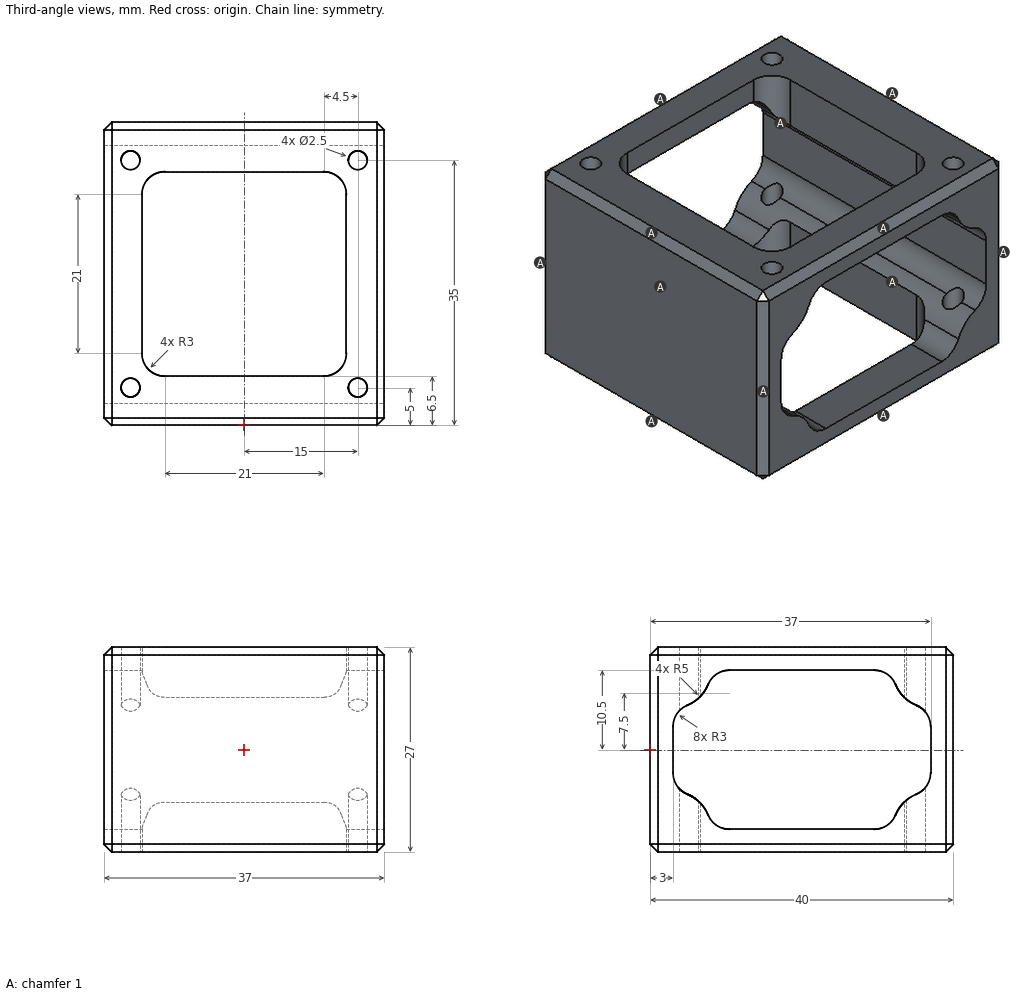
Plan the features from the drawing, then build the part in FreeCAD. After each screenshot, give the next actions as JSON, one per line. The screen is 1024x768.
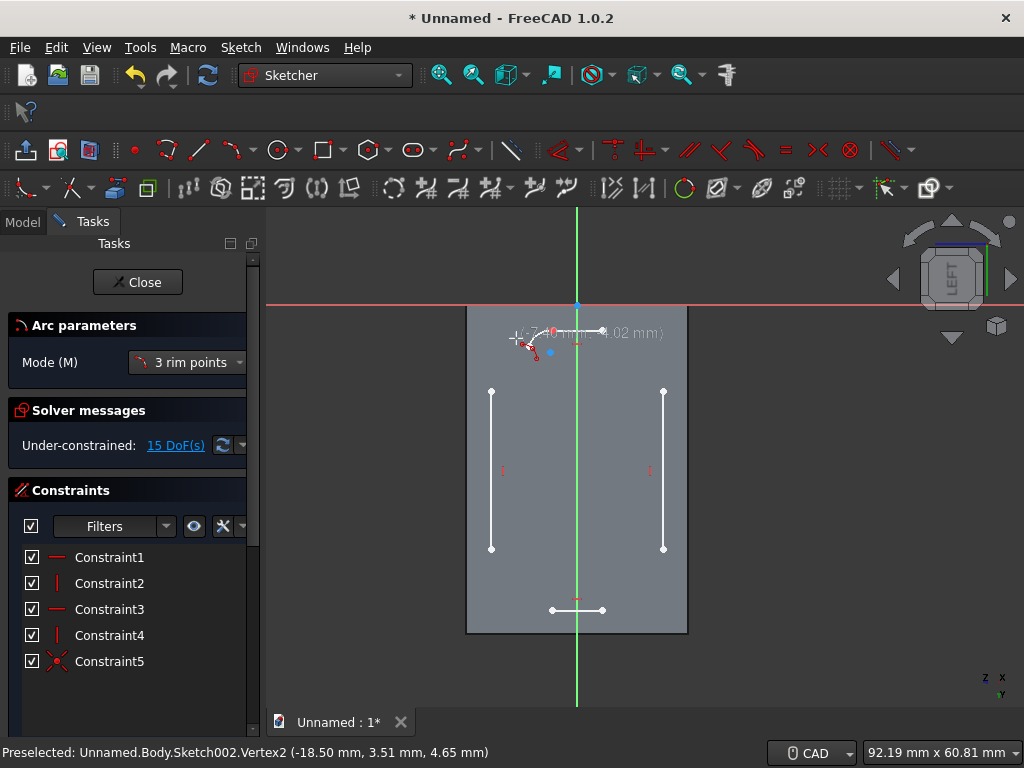
{"action": "left_click", "coordinate": [529, 347]}
{"action": "left_click", "coordinate": [506, 368]}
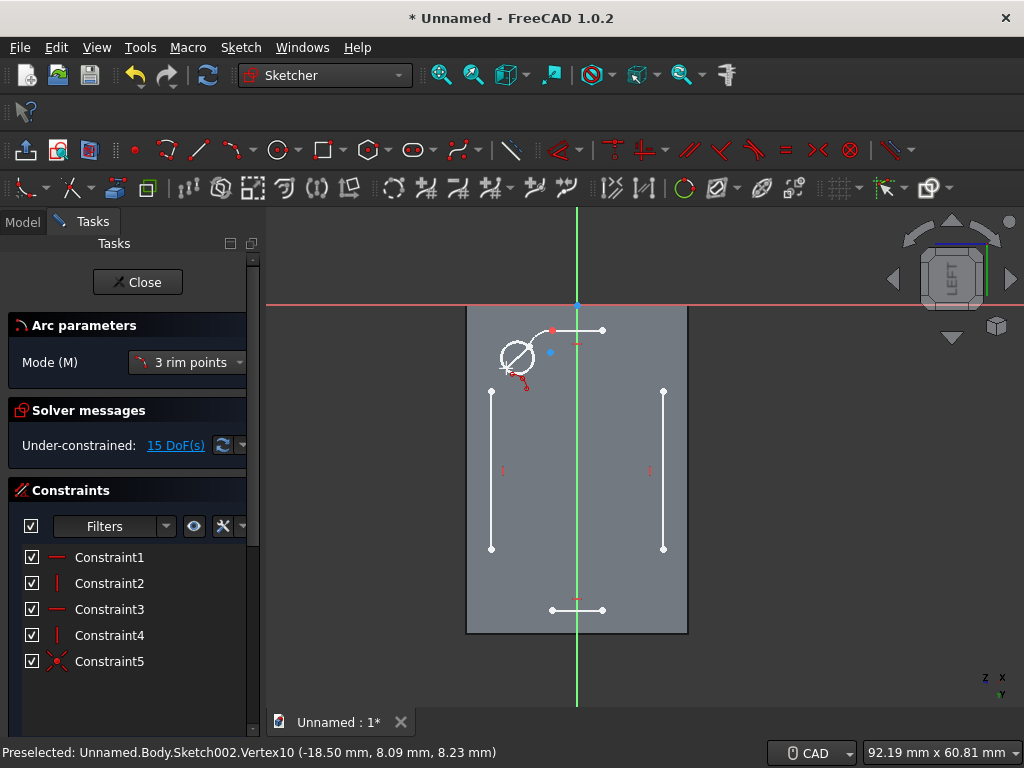
{"action": "scroll", "coordinate": [520, 359], "scroll_direction": "up", "scroll_amount": 8}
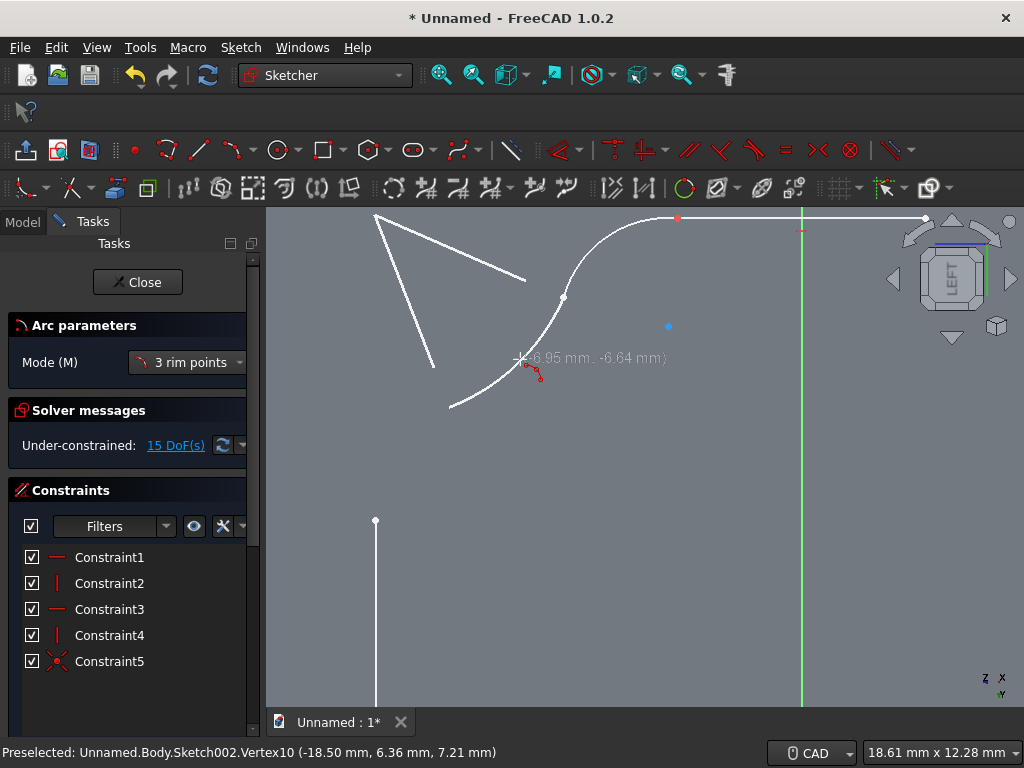
{"action": "left_click", "coordinate": [518, 358]}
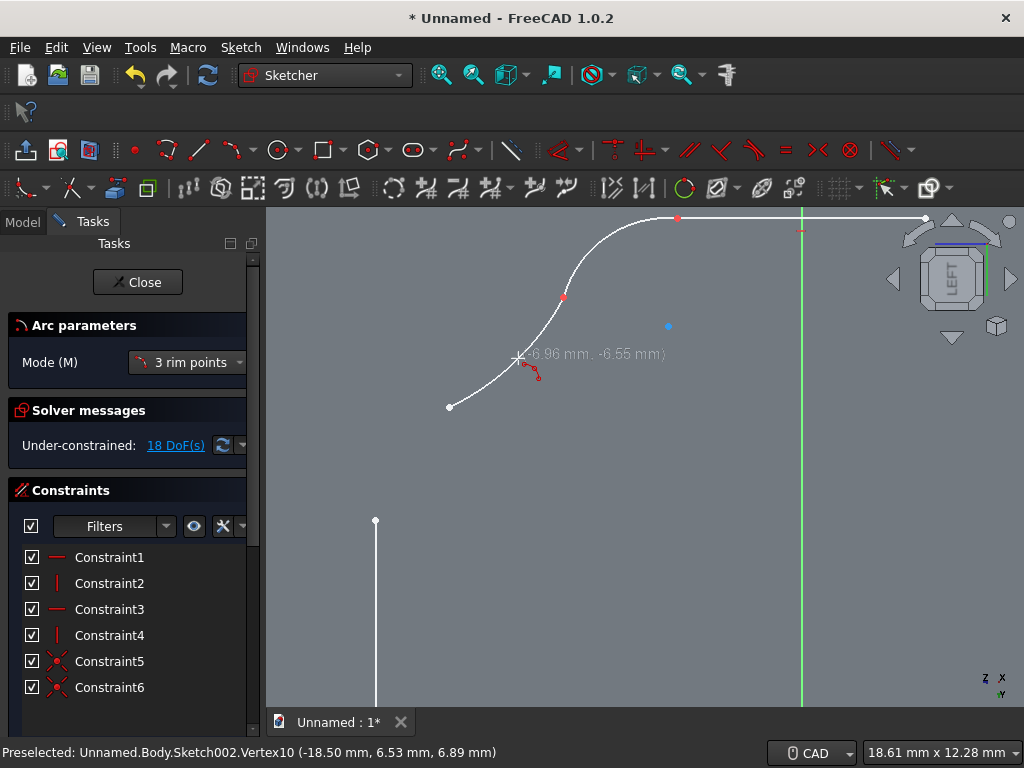
{"action": "scroll", "coordinate": [520, 359], "scroll_direction": "down", "scroll_amount": 8}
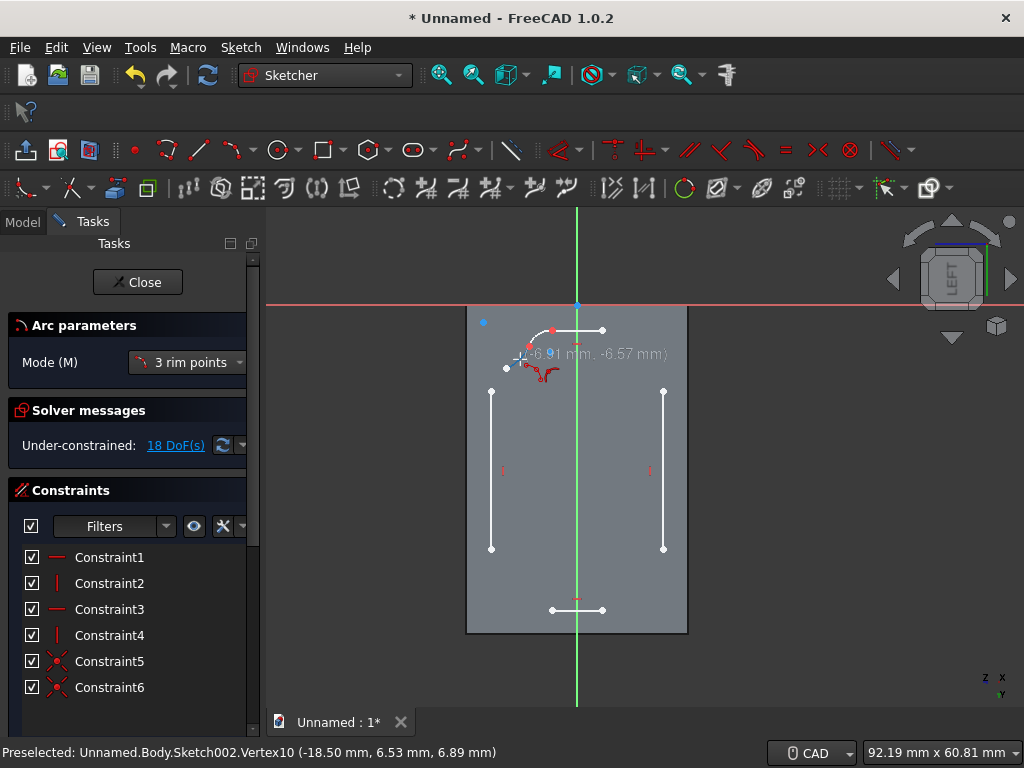
{"action": "left_click", "coordinate": [506, 369]}
{"action": "left_click", "coordinate": [491, 392]}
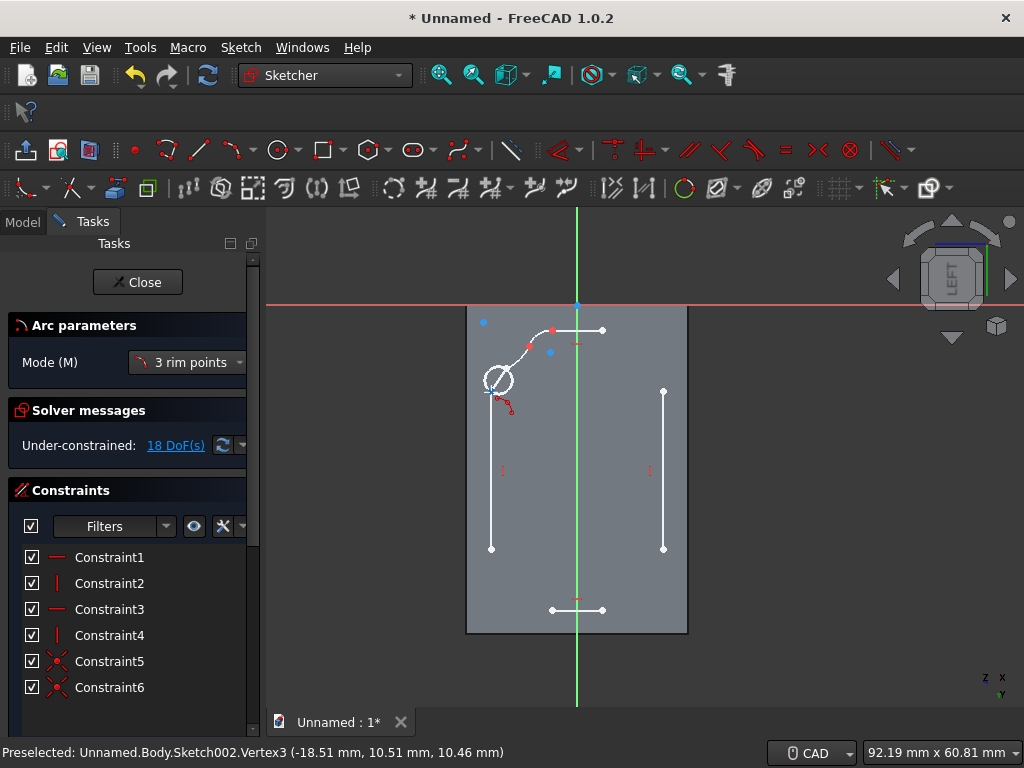
{"action": "scroll", "coordinate": [495, 377], "scroll_direction": "up", "scroll_amount": 7}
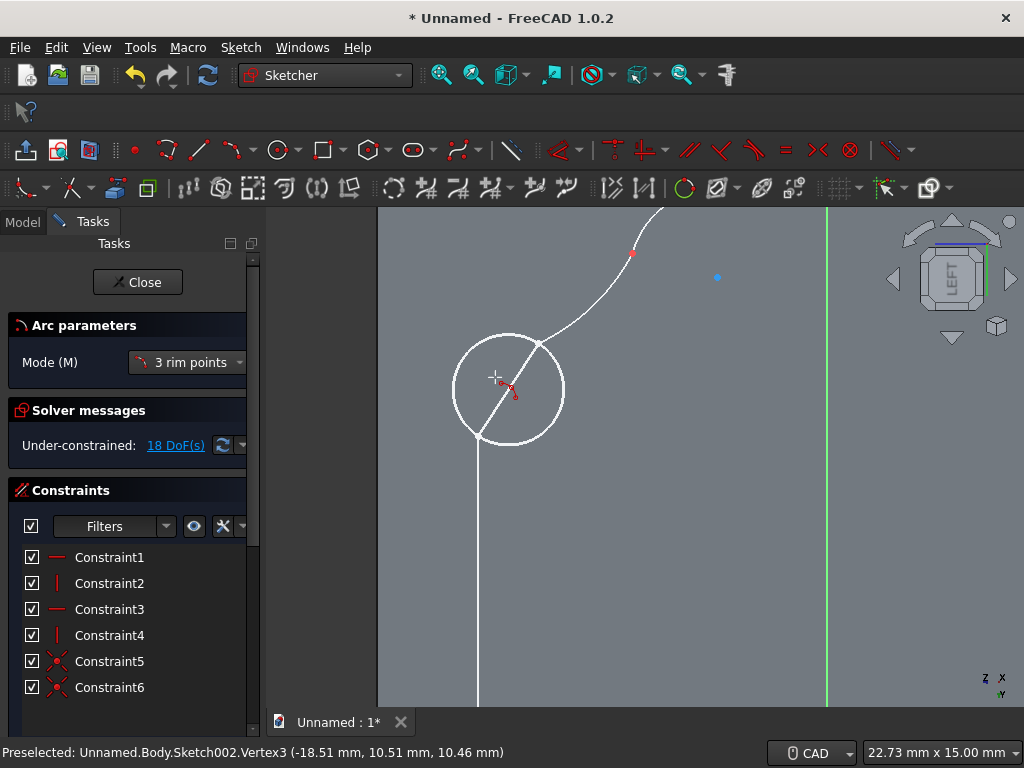
{"action": "left_click", "coordinate": [494, 377]}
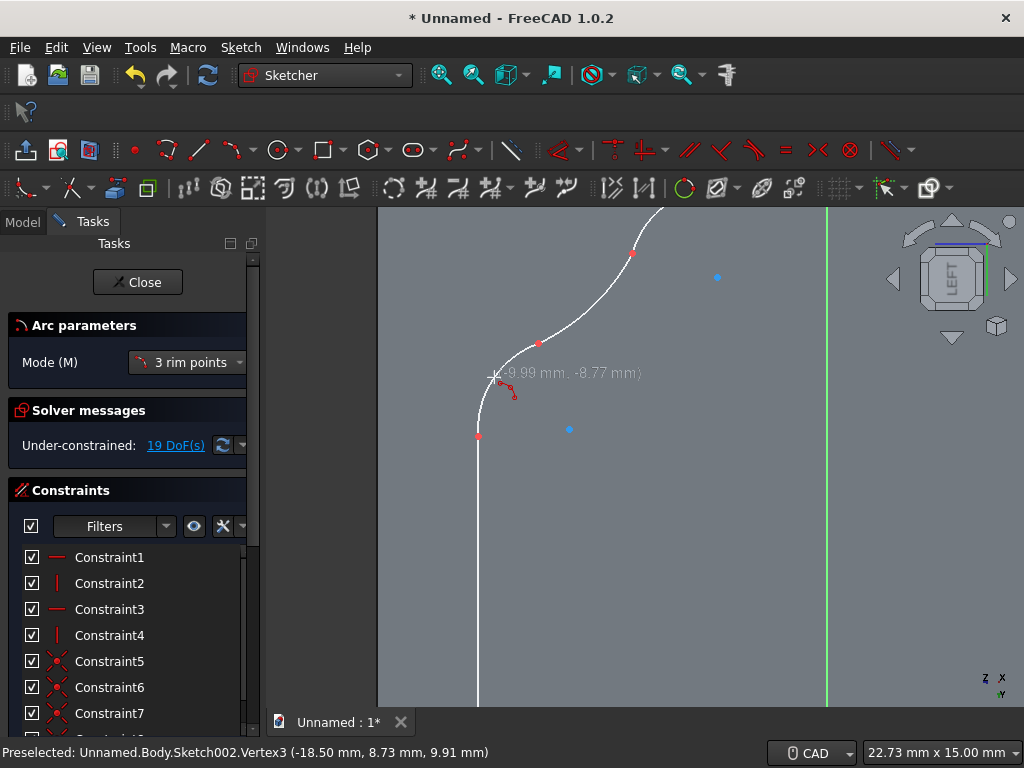
{"action": "scroll", "coordinate": [495, 377], "scroll_direction": "down", "scroll_amount": 7}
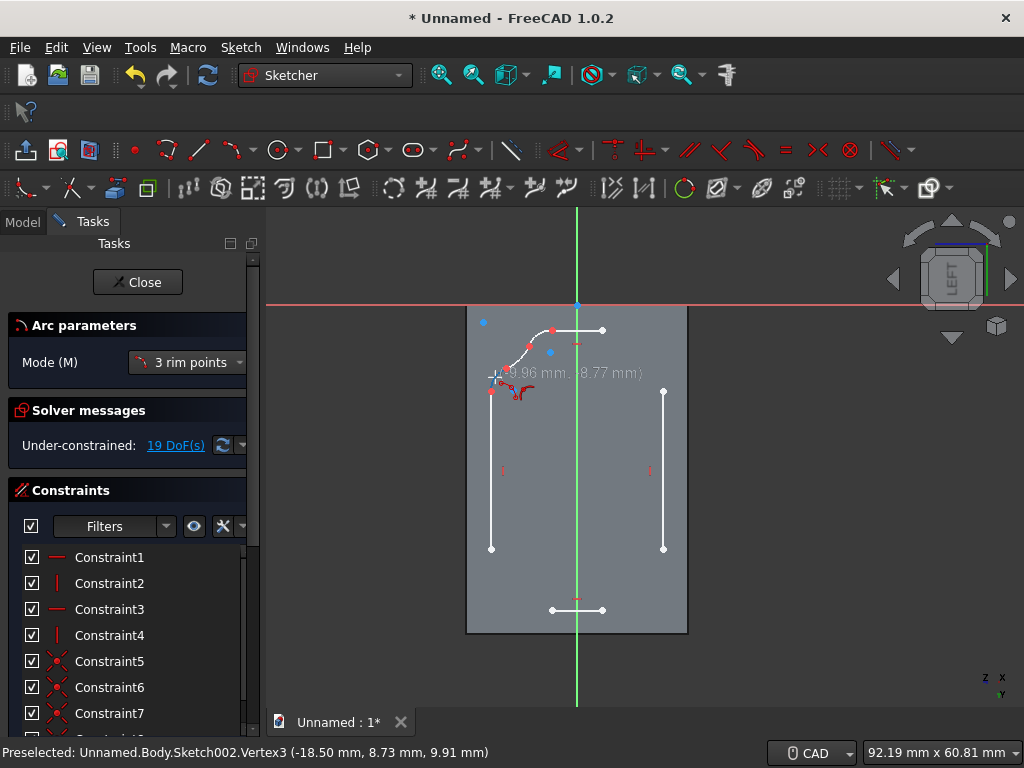
{"action": "left_click", "coordinate": [491, 550]}
{"action": "left_click", "coordinate": [506, 571]}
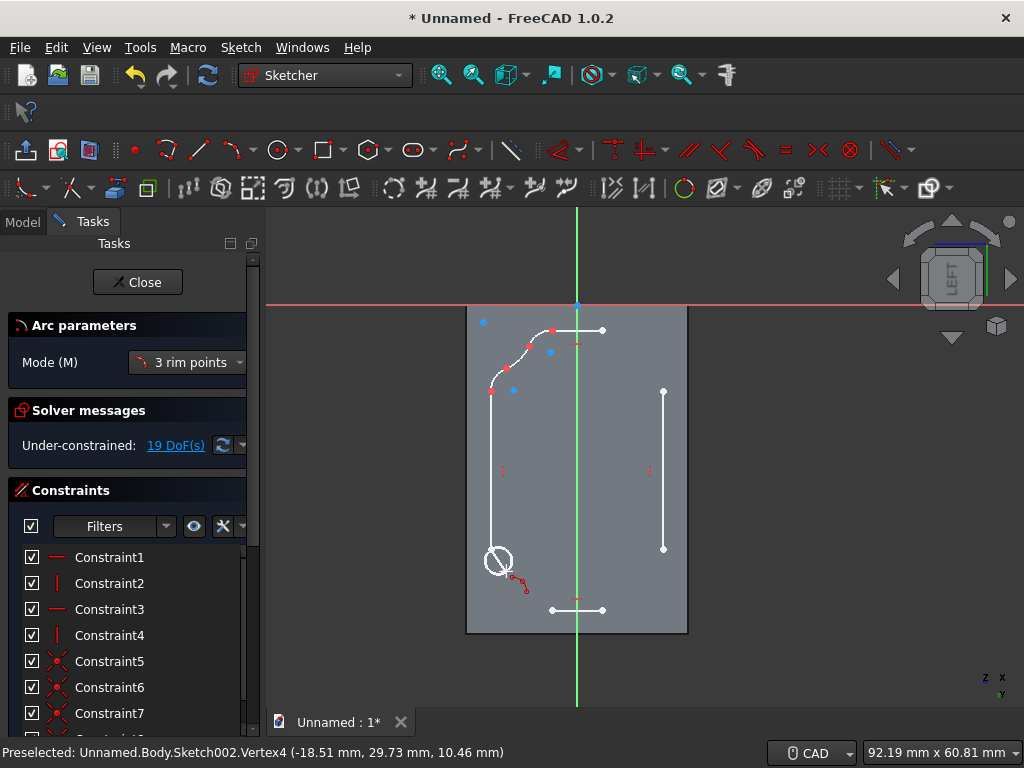
{"action": "scroll", "coordinate": [495, 562], "scroll_direction": "up", "scroll_amount": 7}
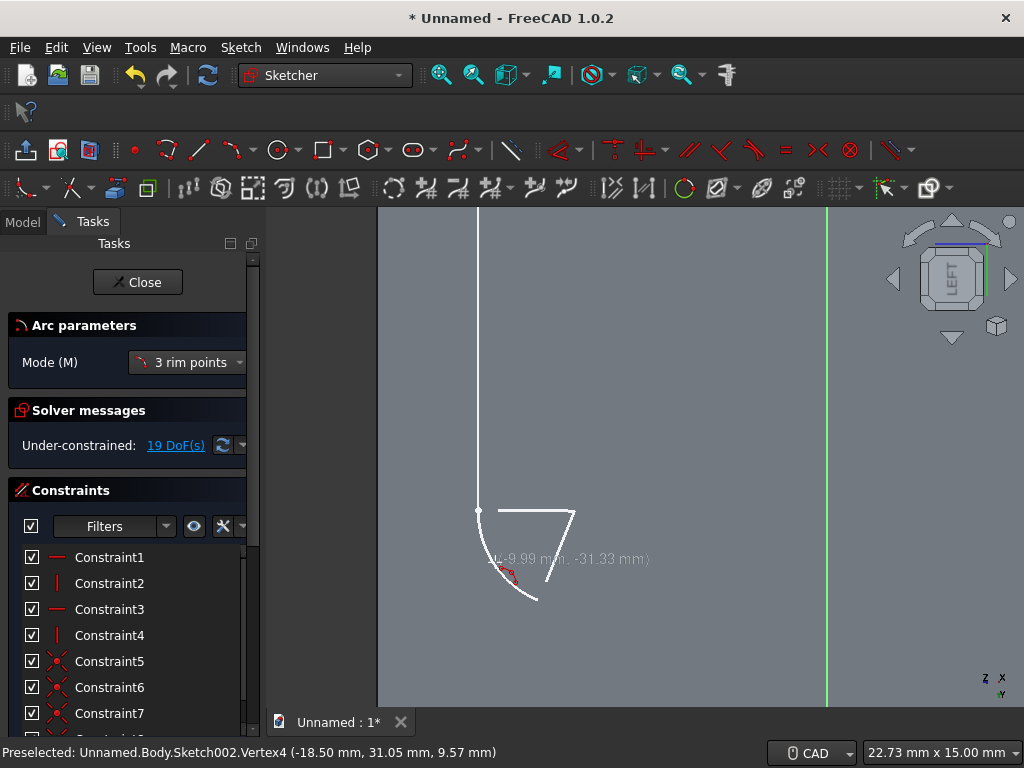
{"action": "left_click", "coordinate": [494, 562]}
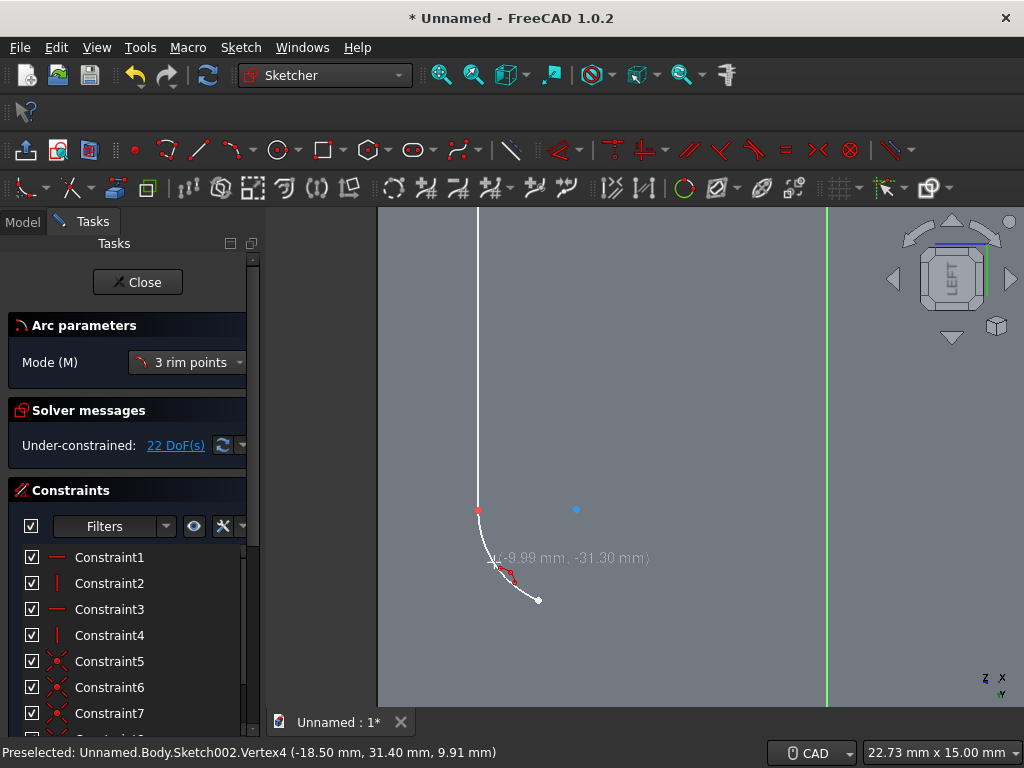
{"action": "scroll", "coordinate": [495, 562], "scroll_direction": "down", "scroll_amount": 7}